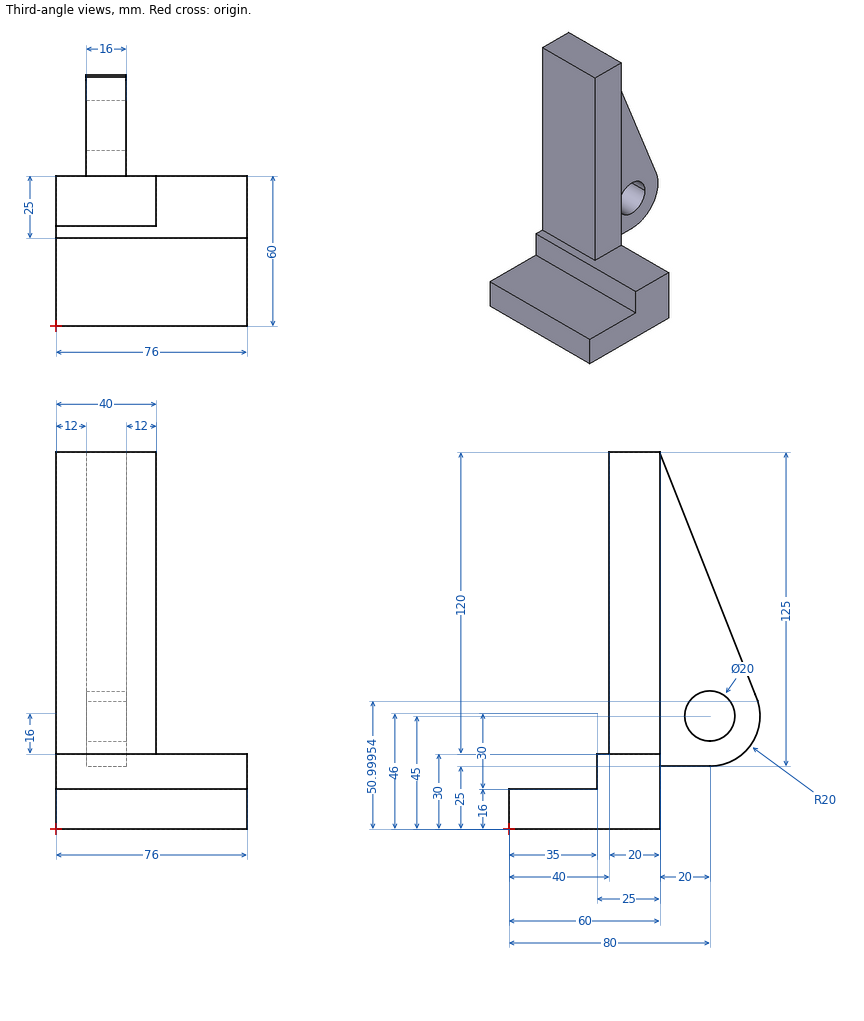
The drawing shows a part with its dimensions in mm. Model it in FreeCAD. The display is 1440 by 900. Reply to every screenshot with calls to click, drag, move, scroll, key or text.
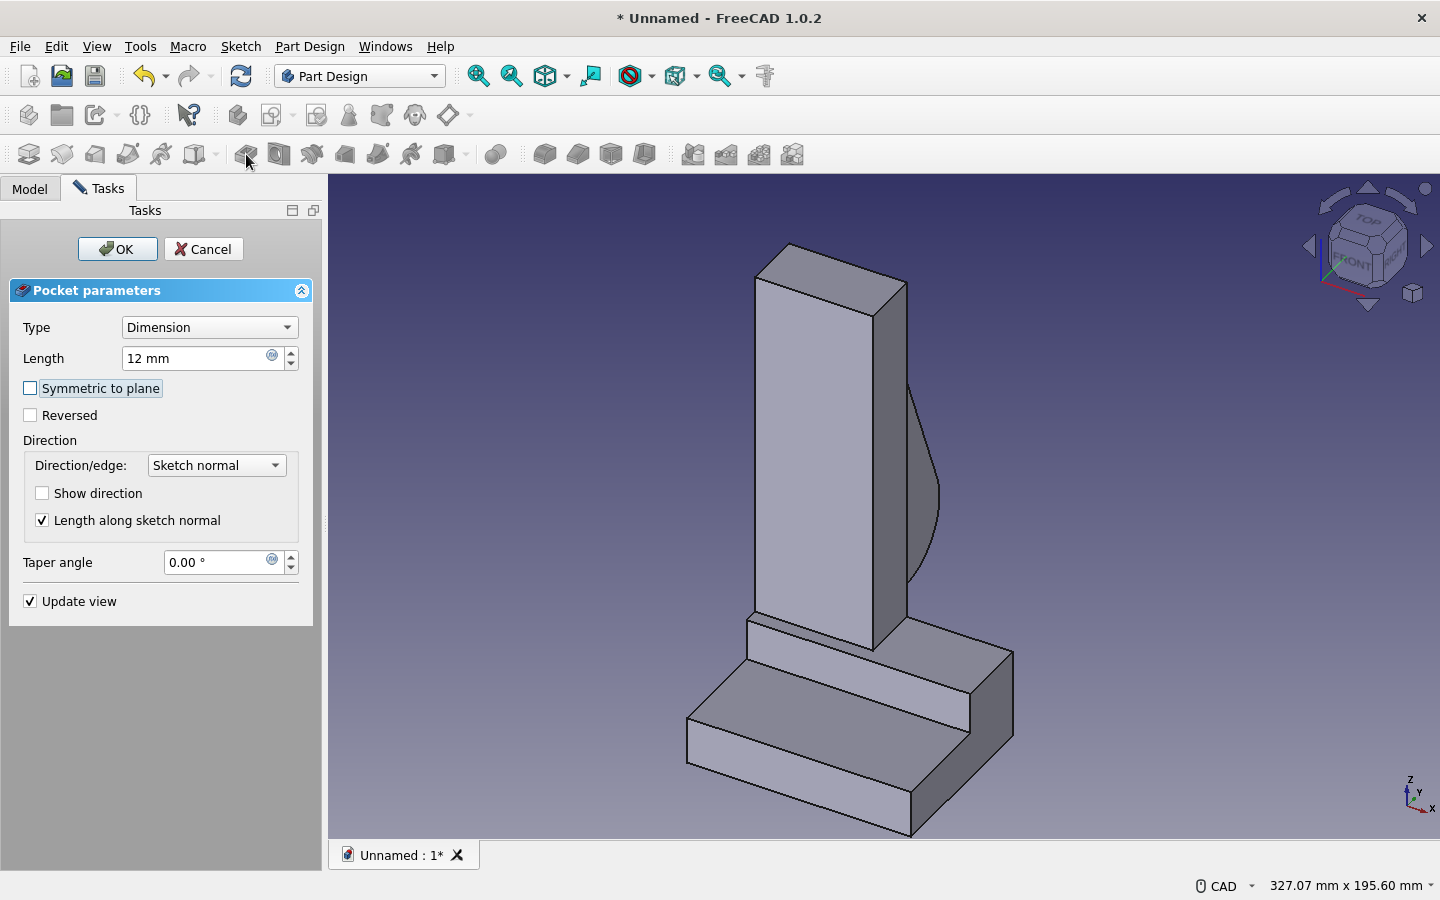
click(118, 249)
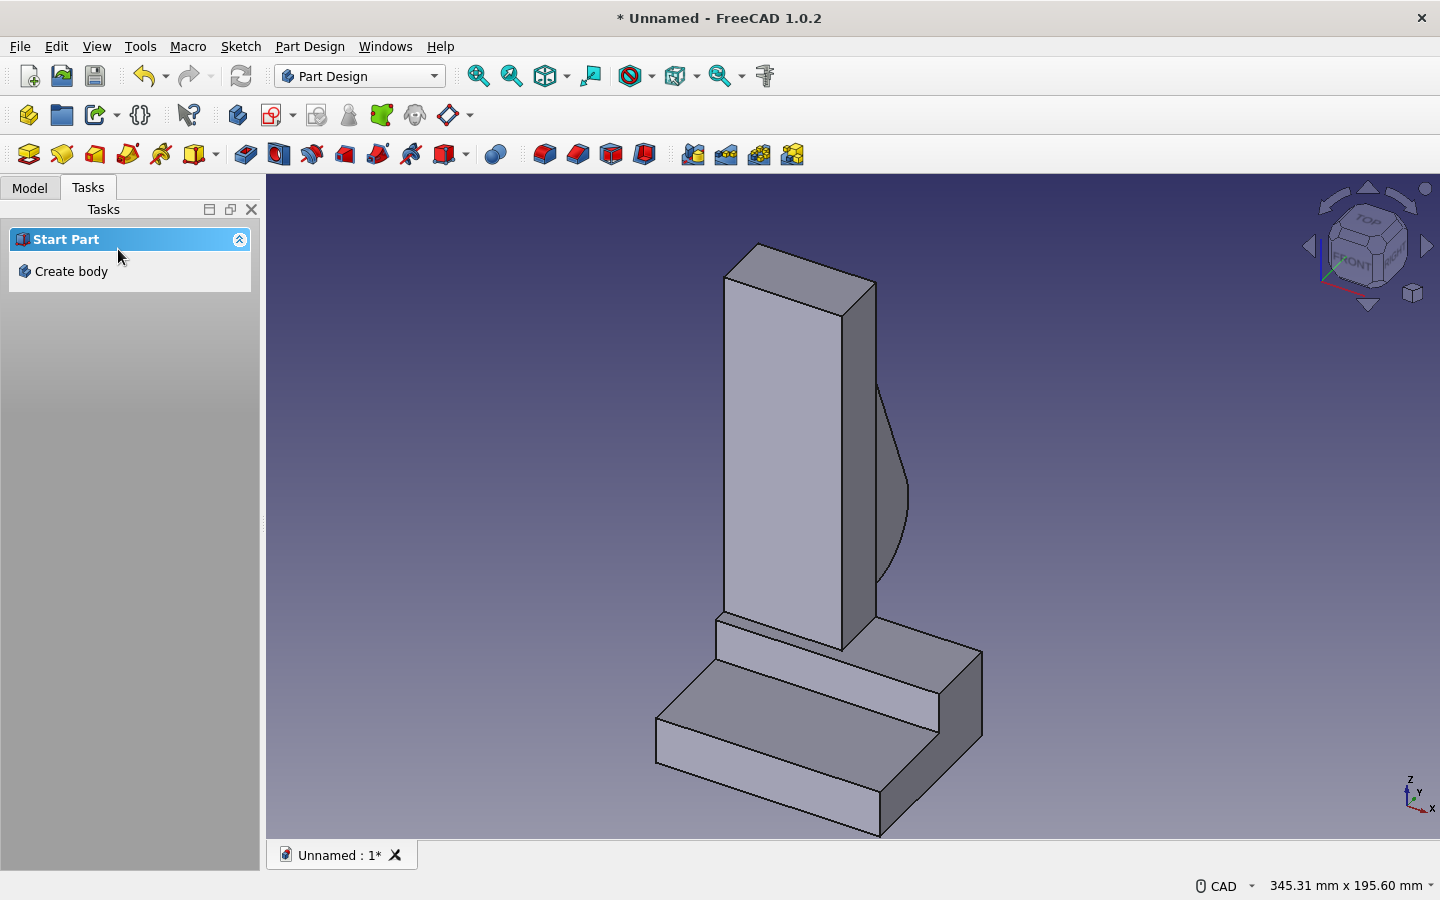
click(30, 188)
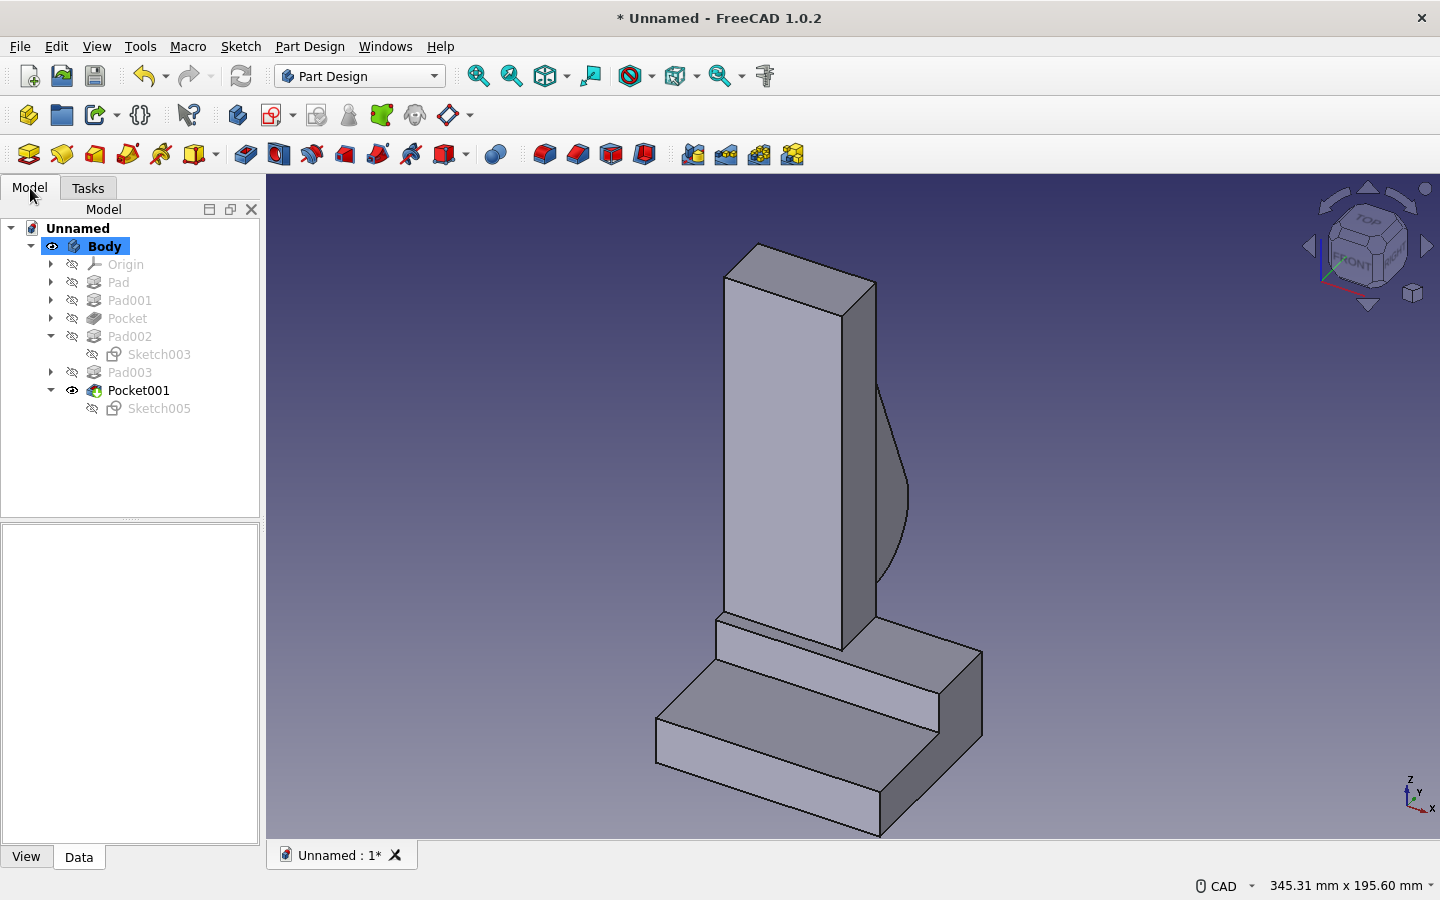
click(51, 264)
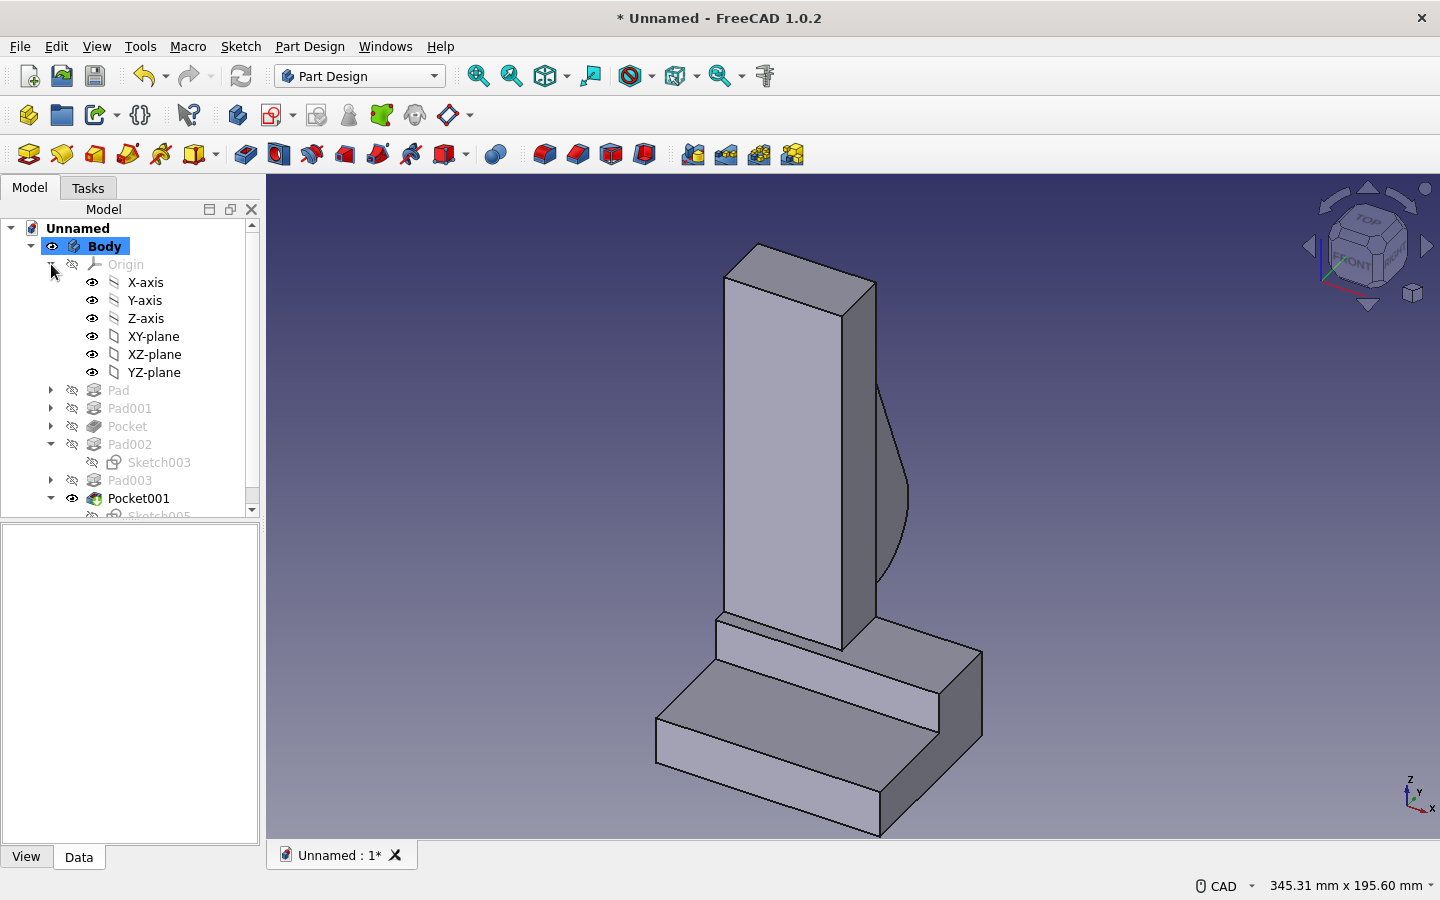
click(137, 372)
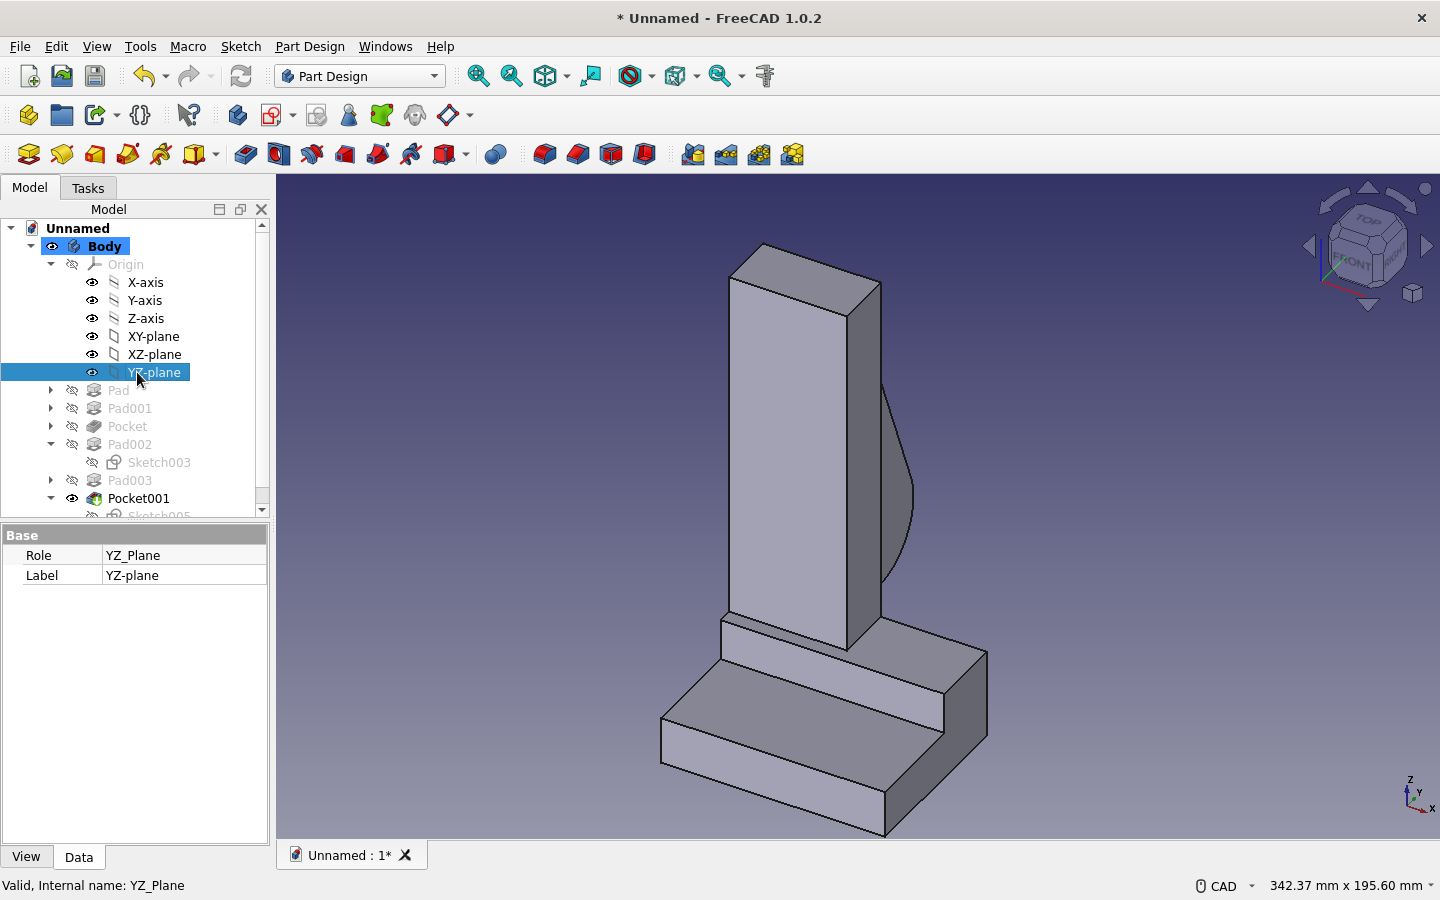
click(448, 116)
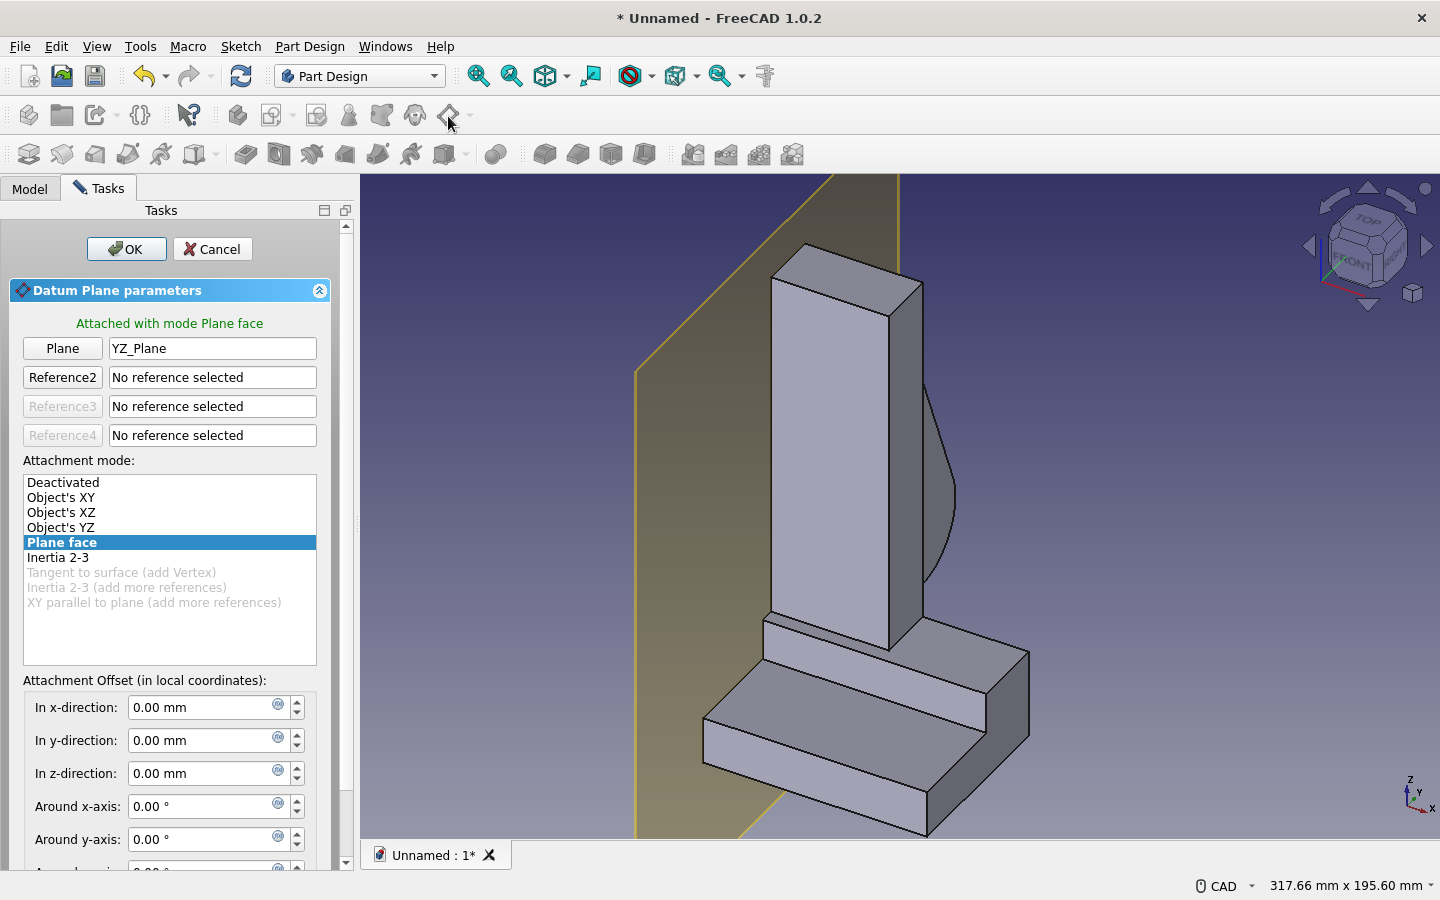
triple_click(210, 774)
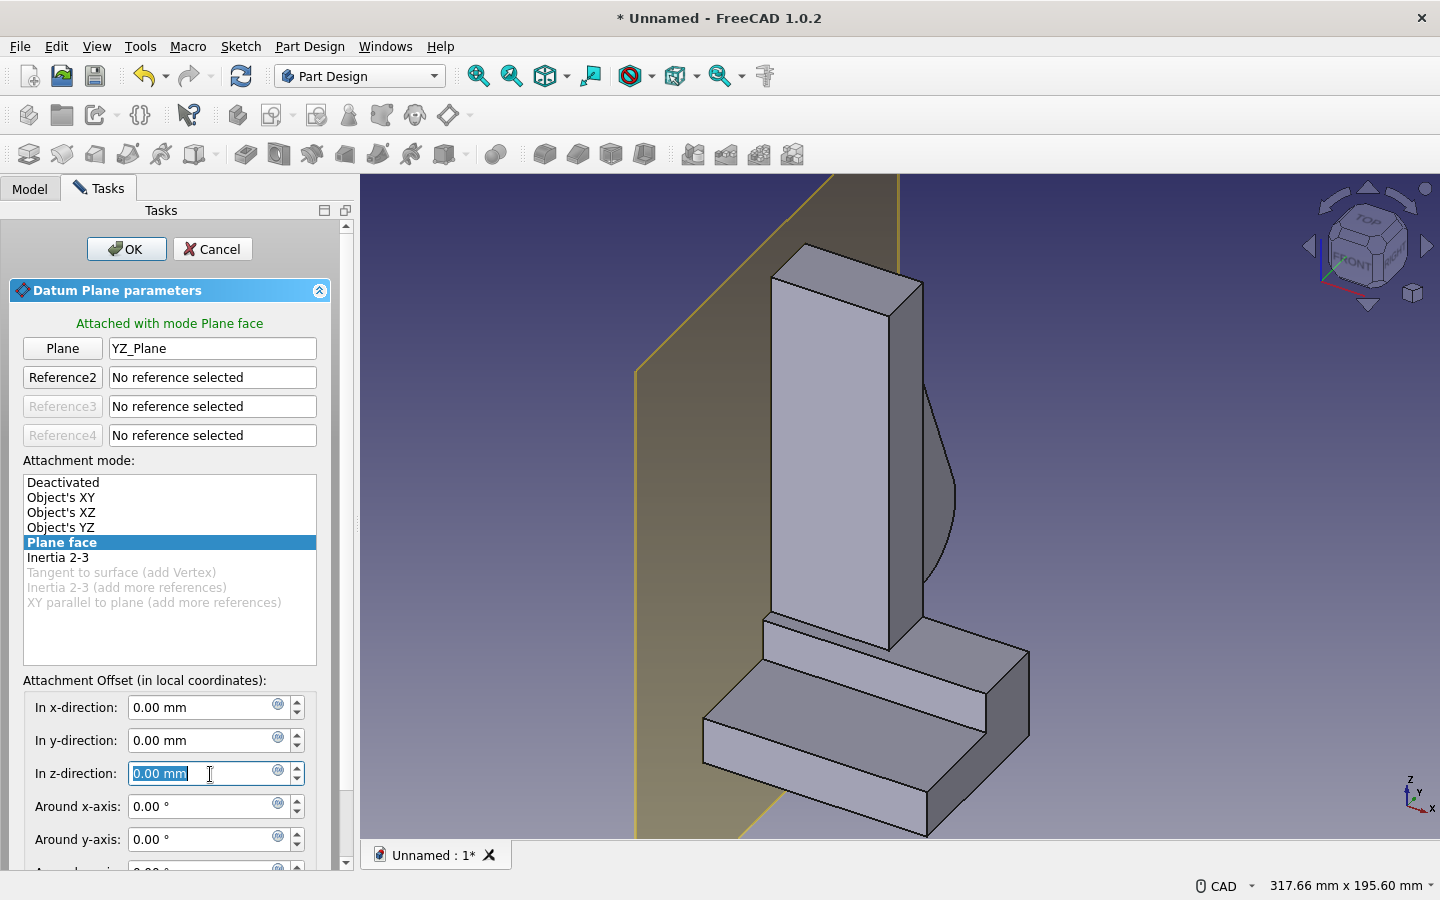
text(12)
key(Tab)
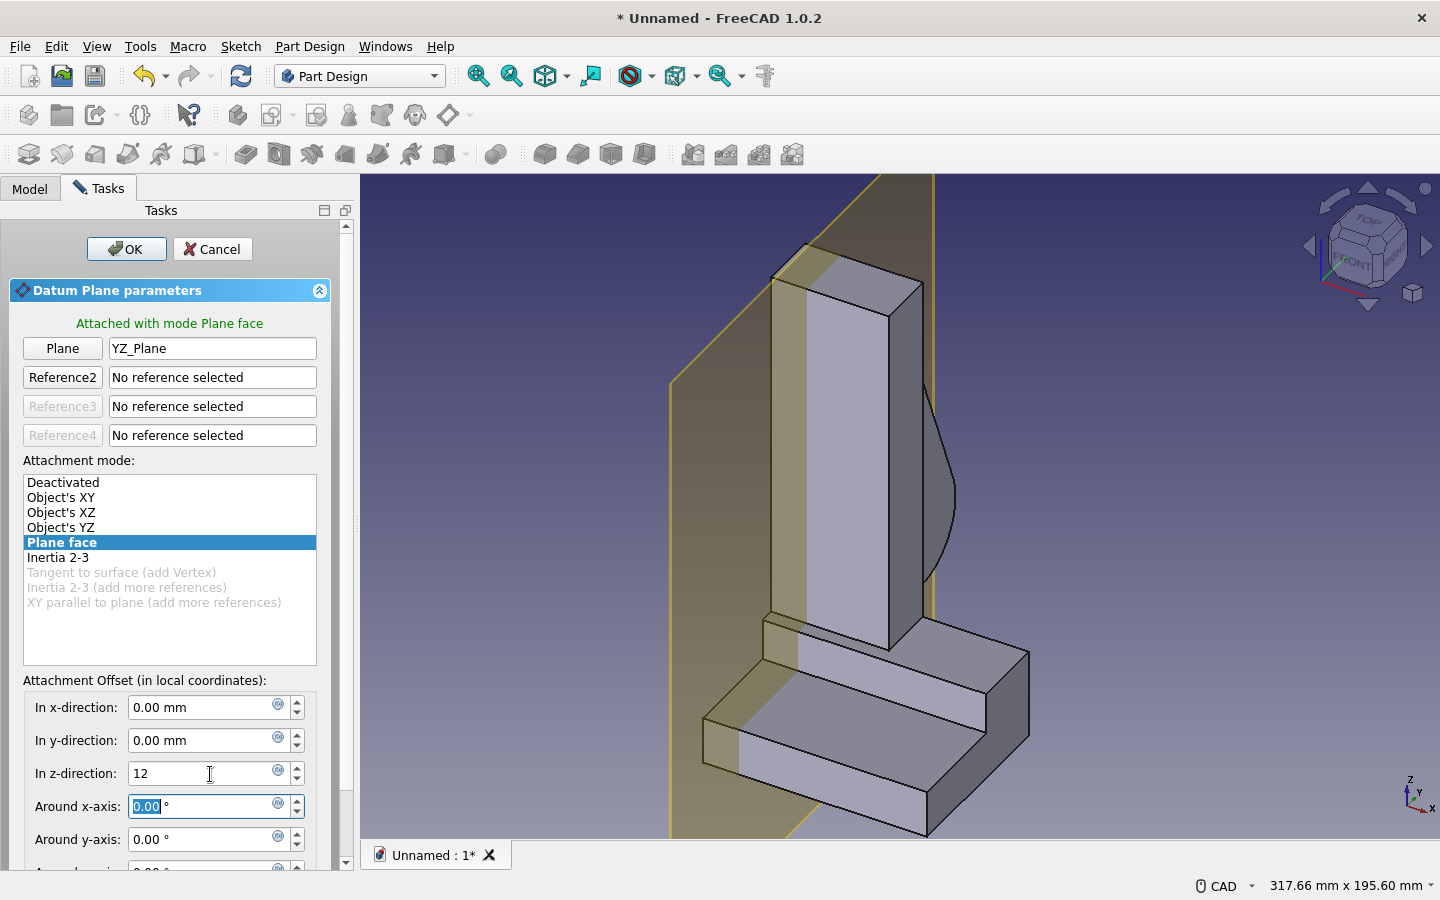
click(127, 249)